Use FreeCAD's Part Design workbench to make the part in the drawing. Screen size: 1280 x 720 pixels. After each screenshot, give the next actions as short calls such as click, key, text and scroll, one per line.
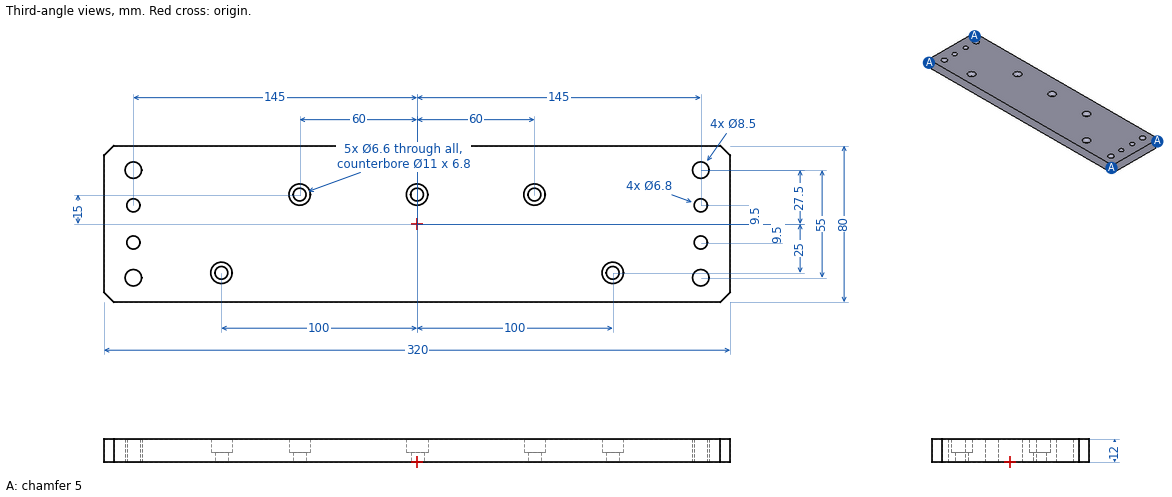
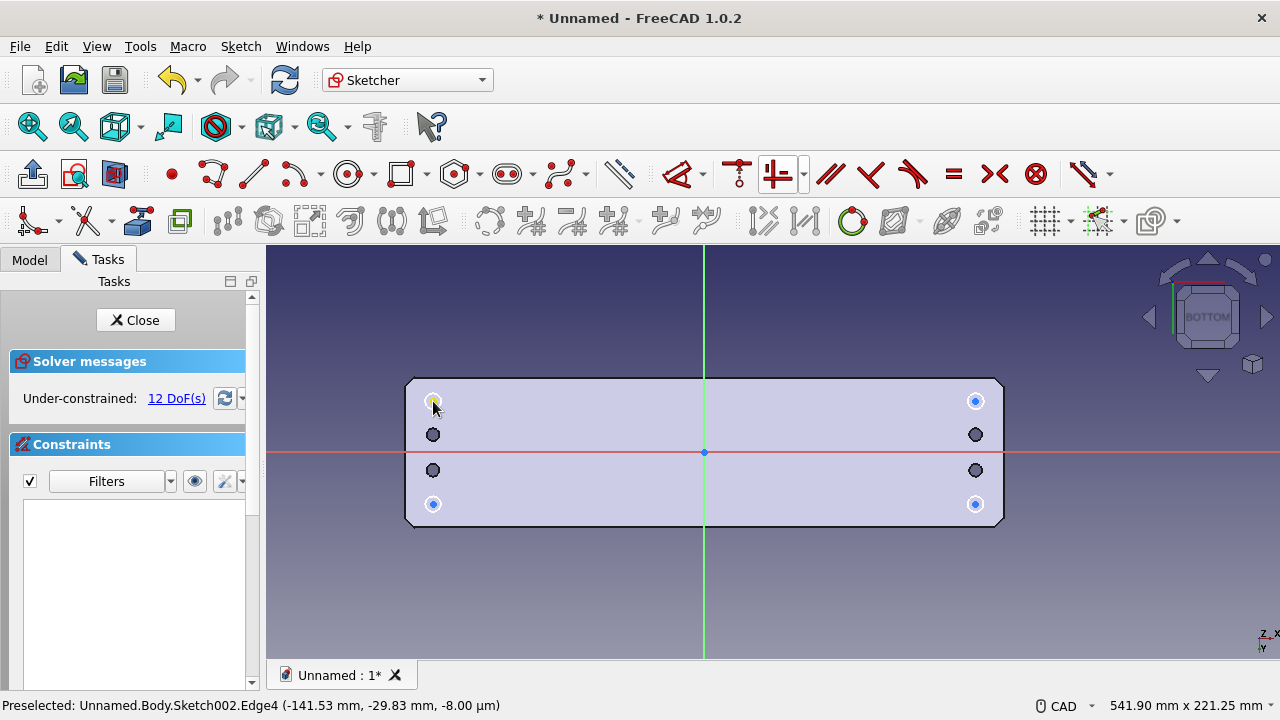
scroll(981, 499, up, 3)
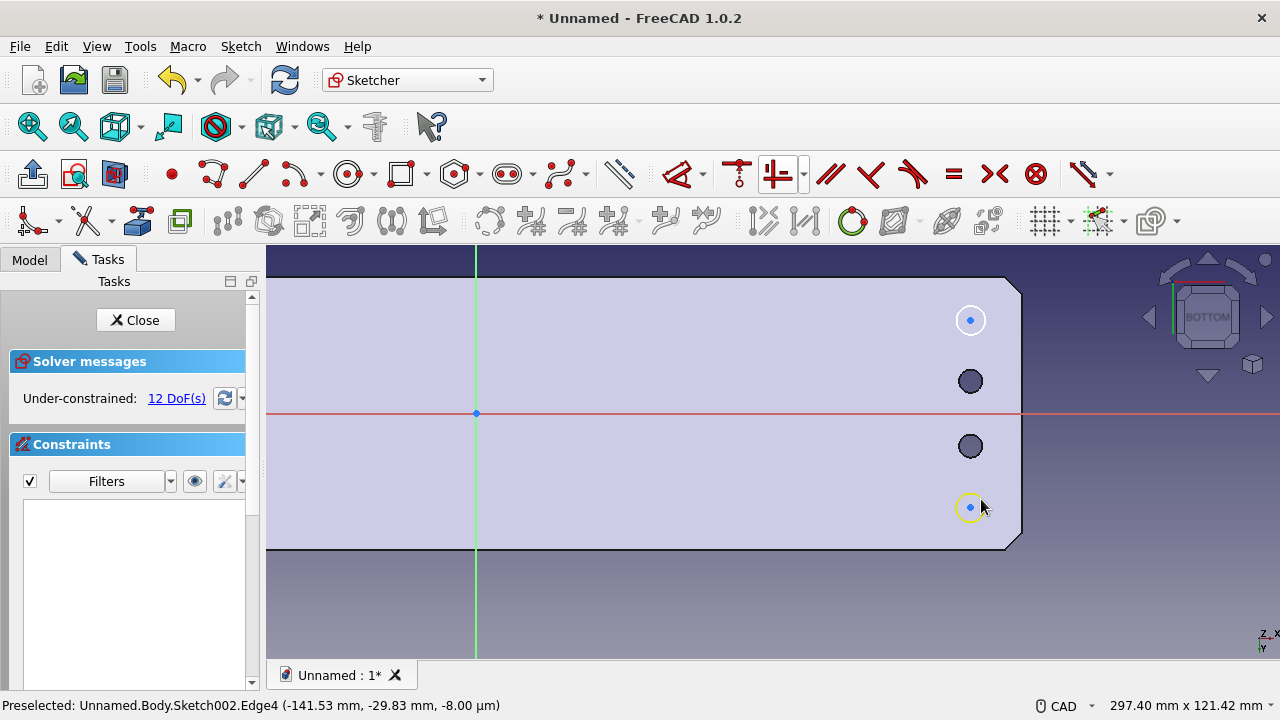
click(981, 498)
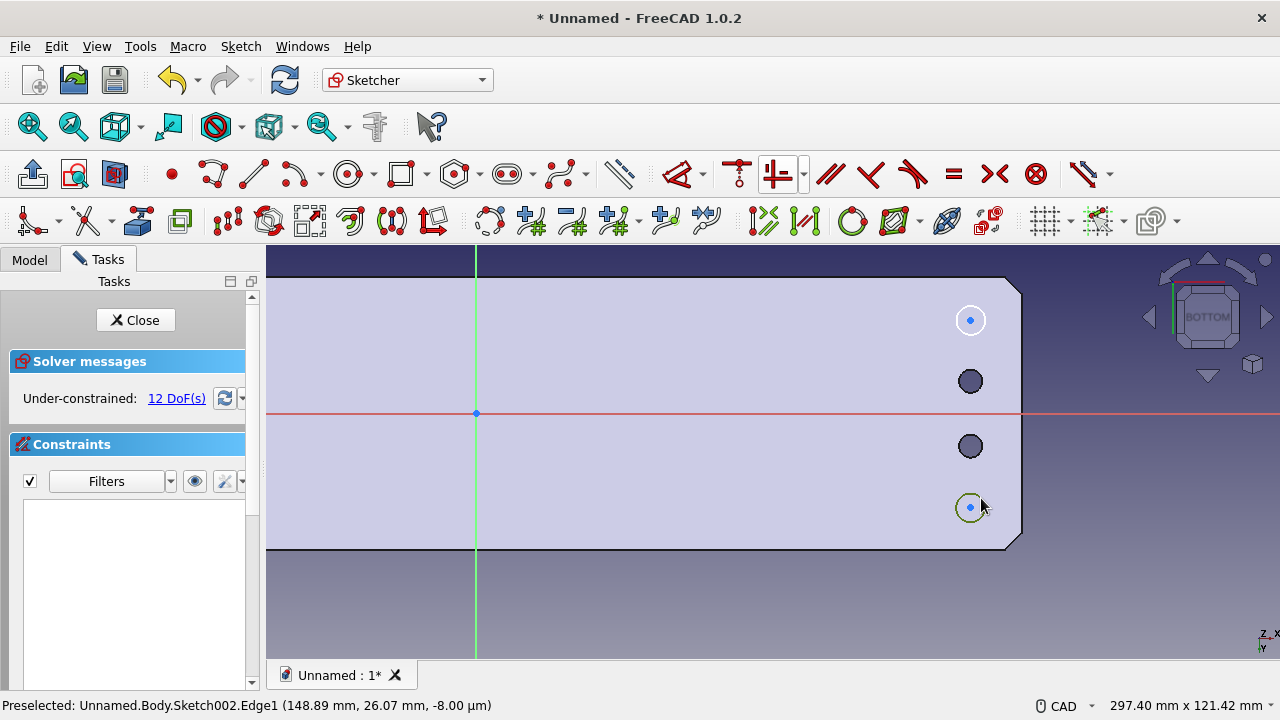
click(981, 310)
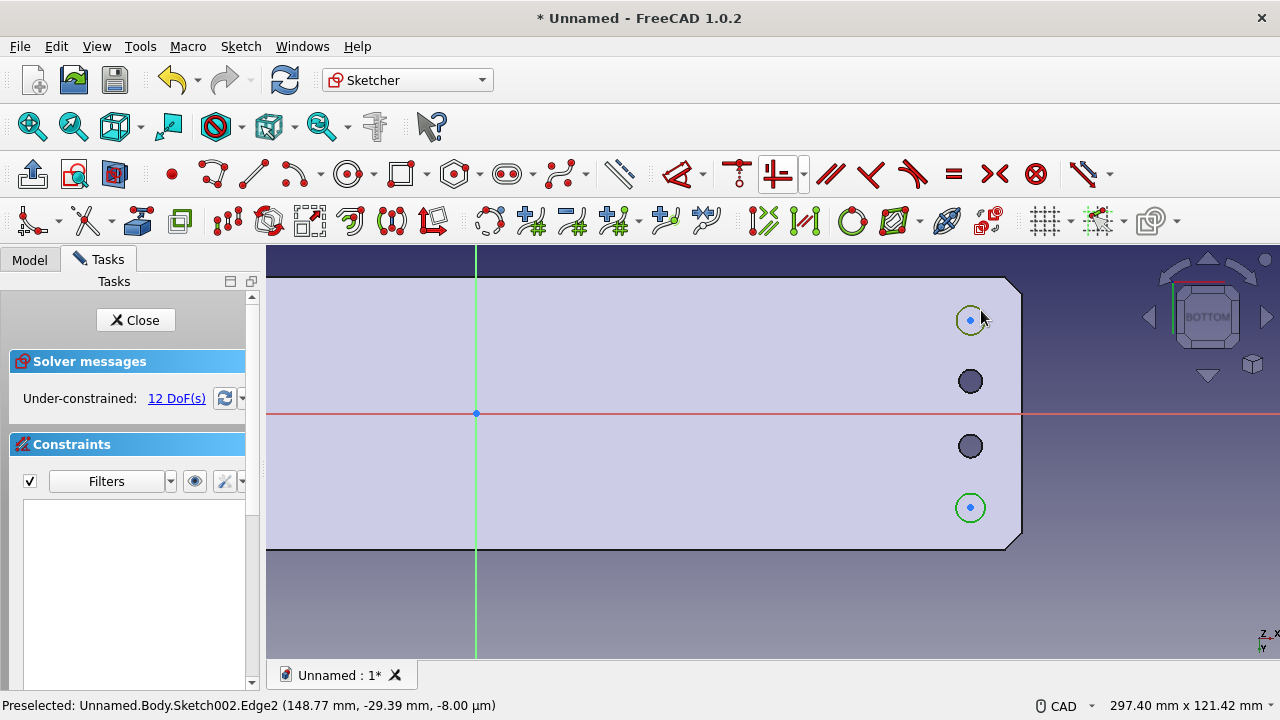
scroll(982, 499, down, 3)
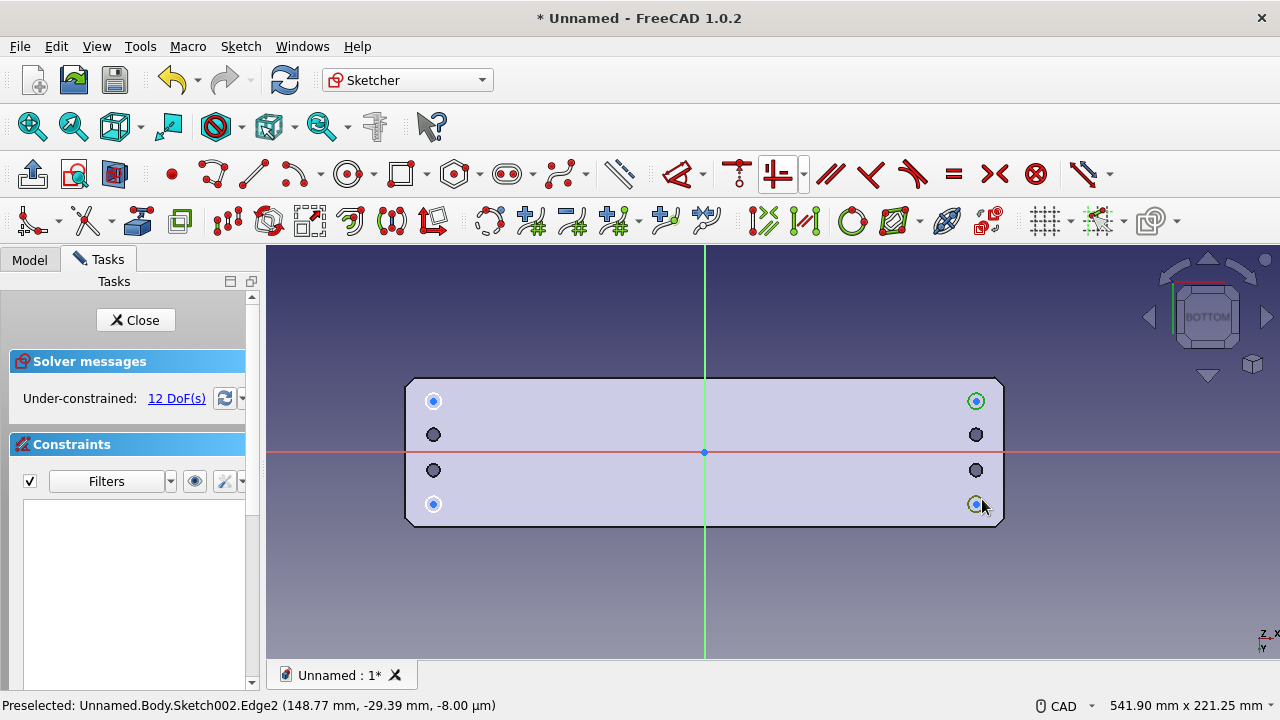
scroll(439, 499, up, 3)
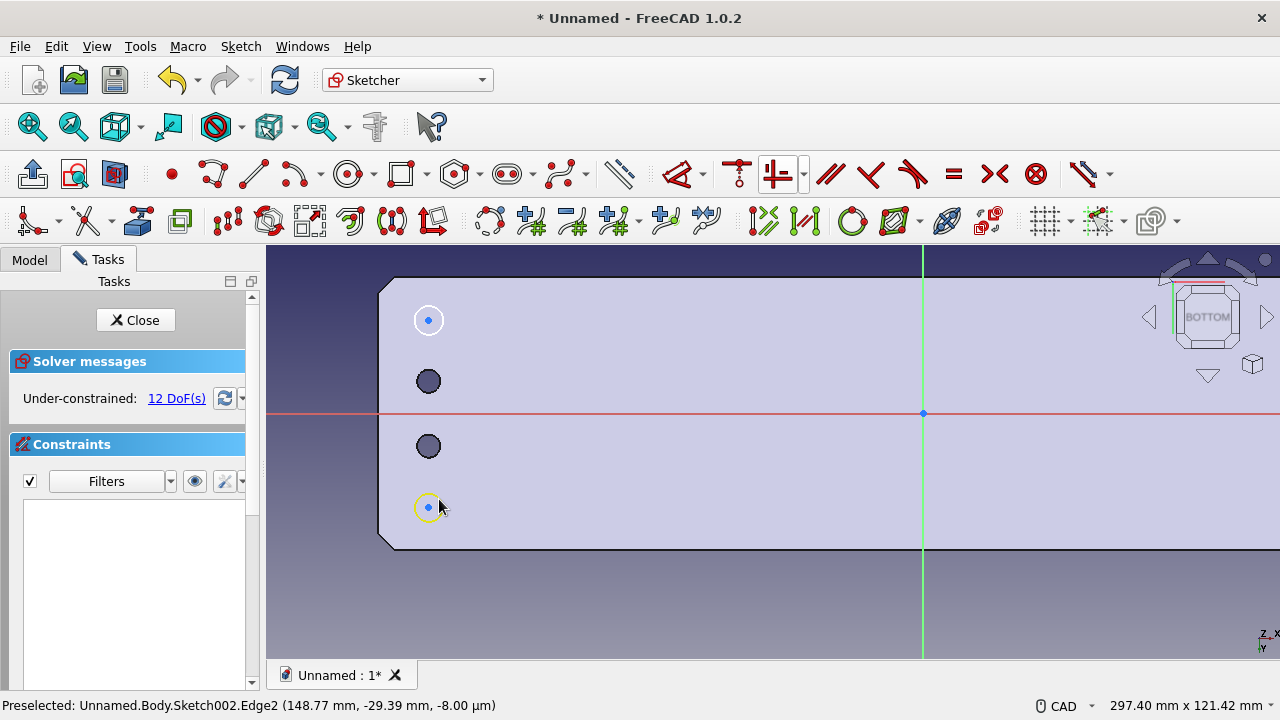
click(439, 498)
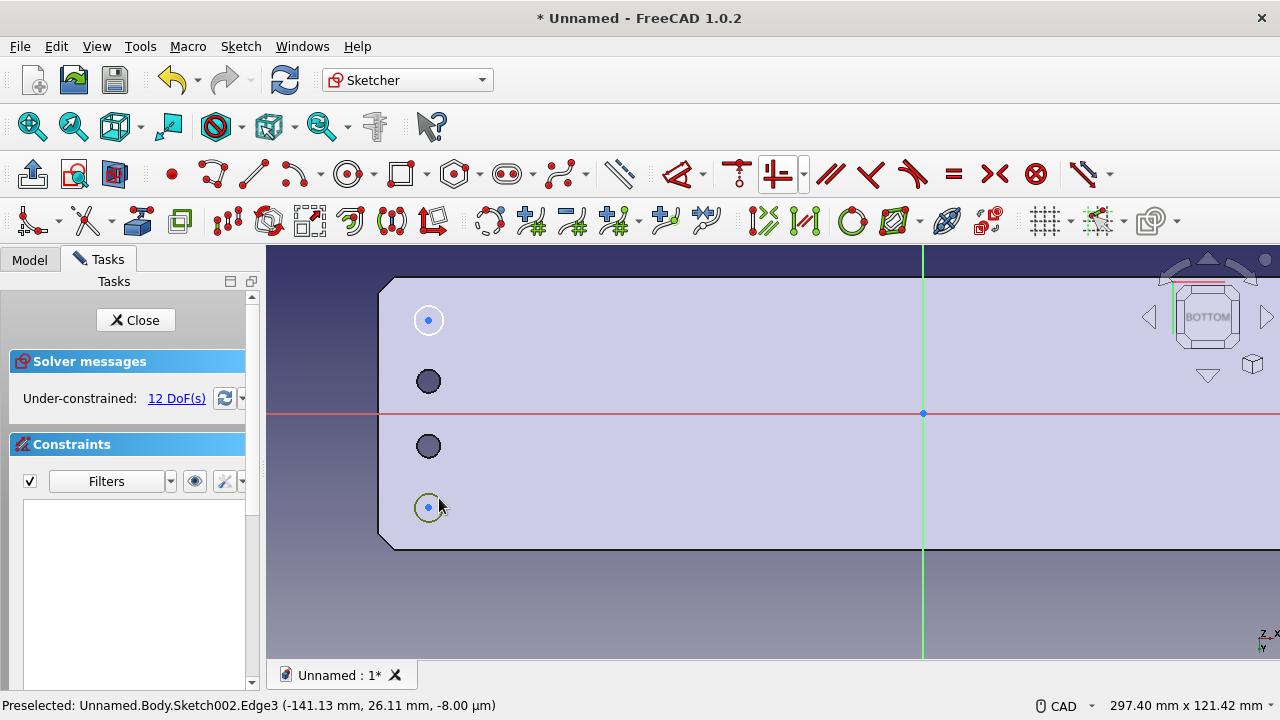
click(439, 310)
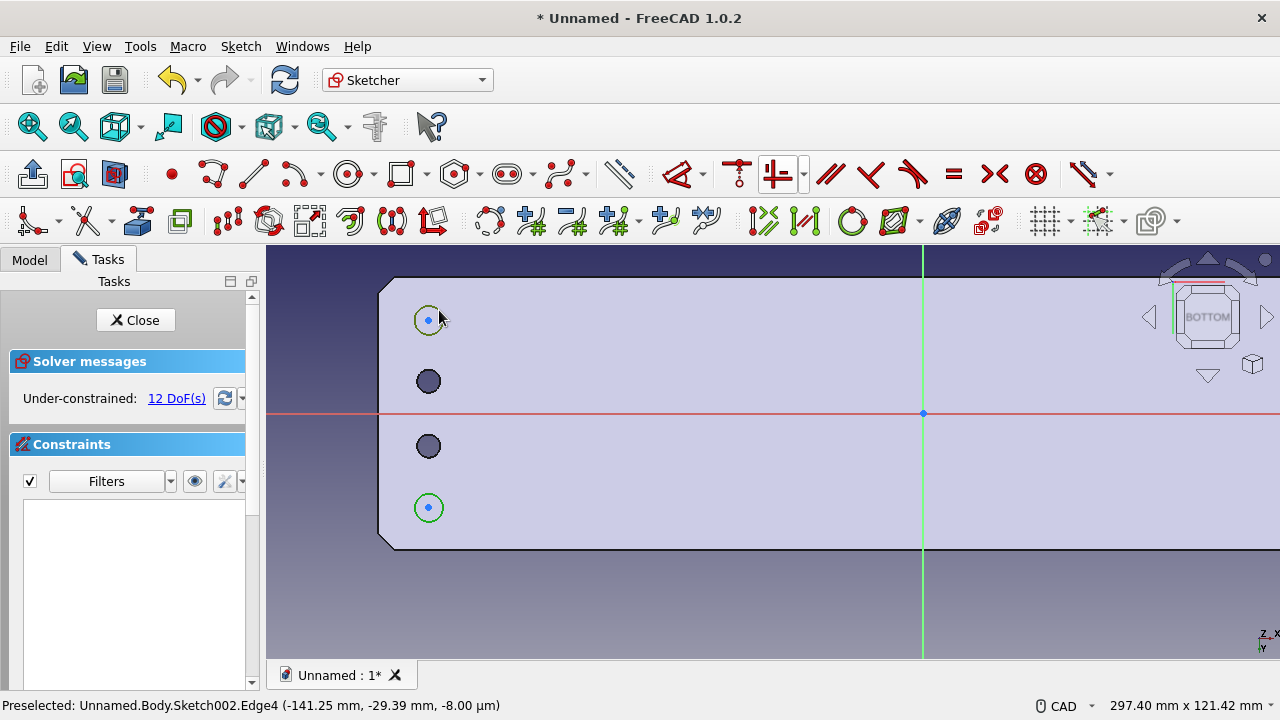
click(954, 174)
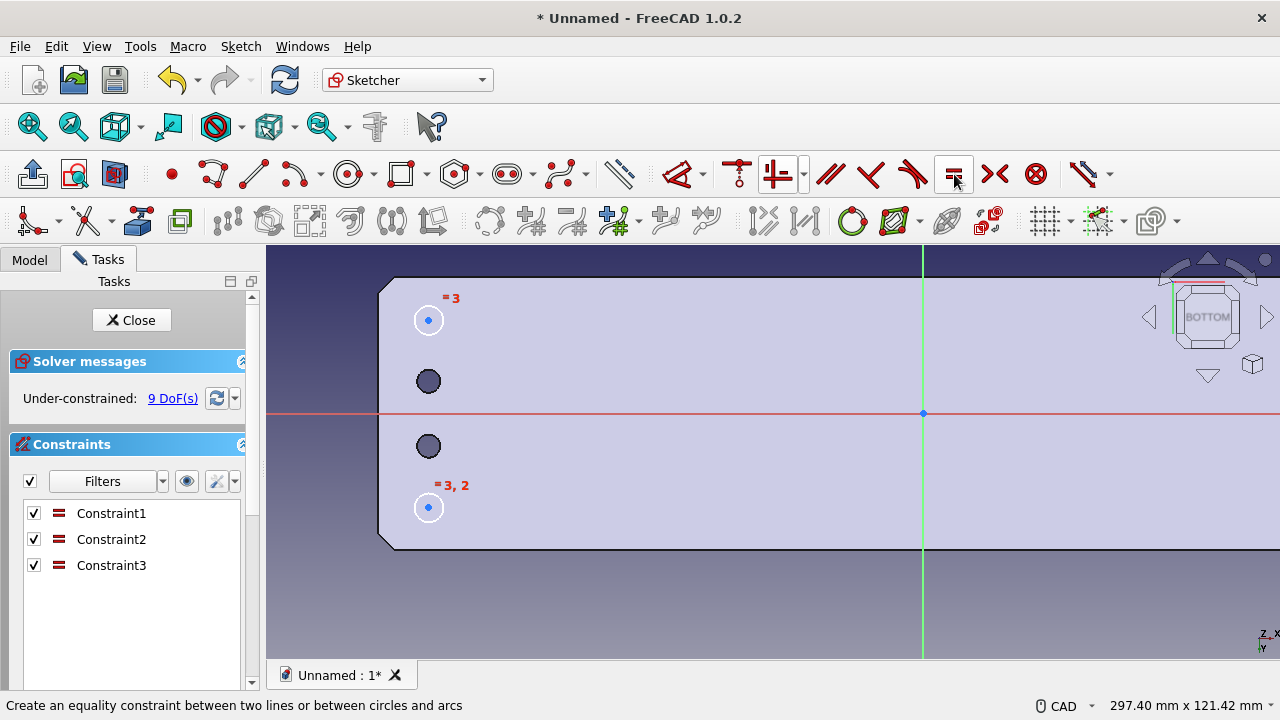
click(676, 174)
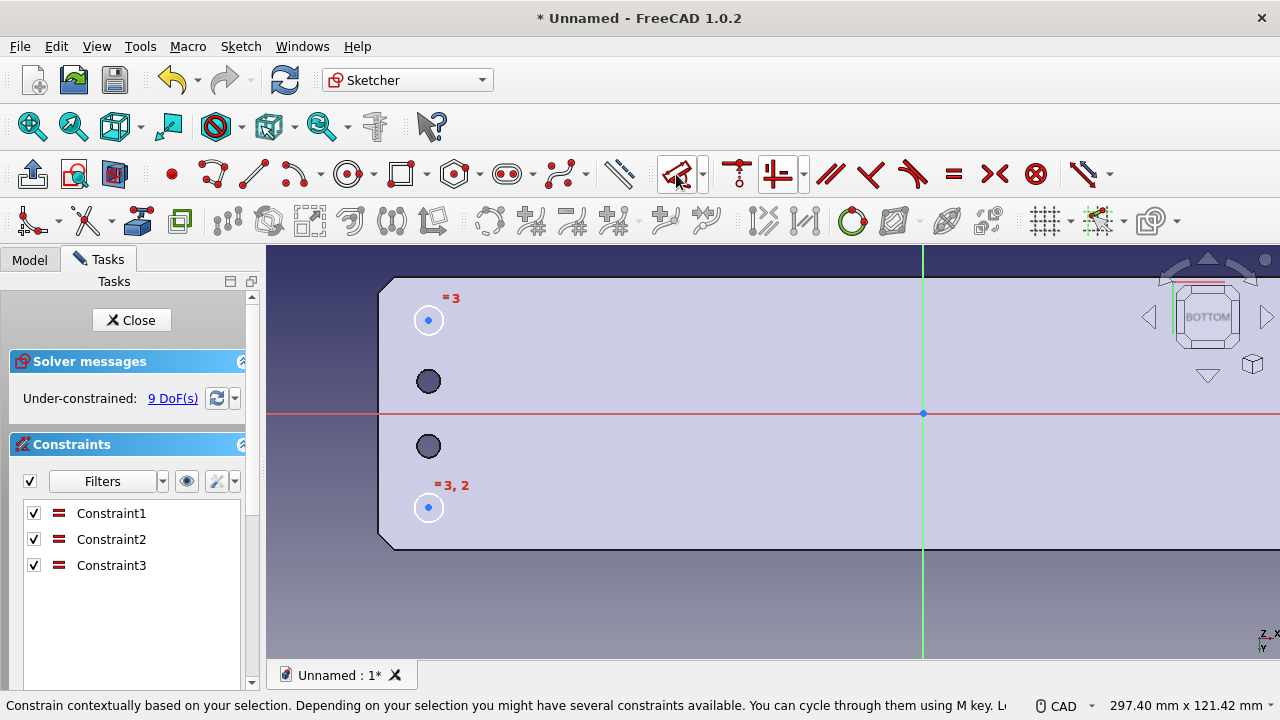
scroll(439, 499, down, 3)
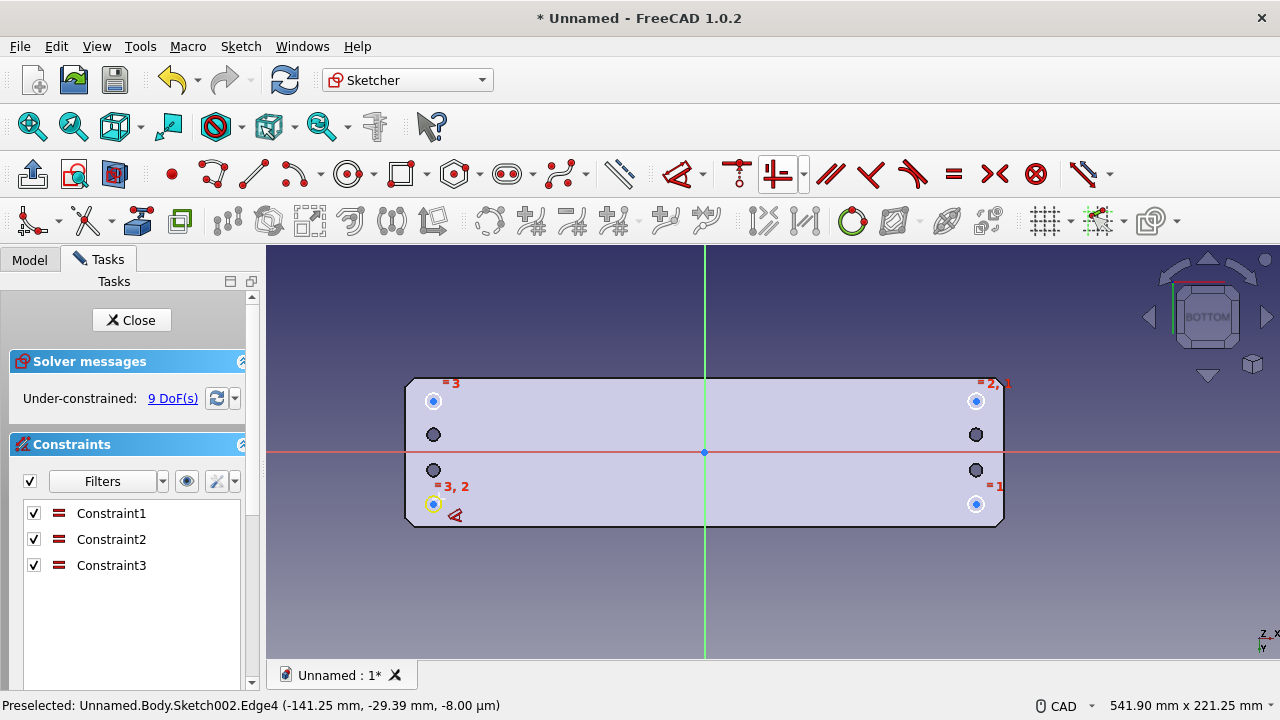
scroll(982, 499, up, 5)